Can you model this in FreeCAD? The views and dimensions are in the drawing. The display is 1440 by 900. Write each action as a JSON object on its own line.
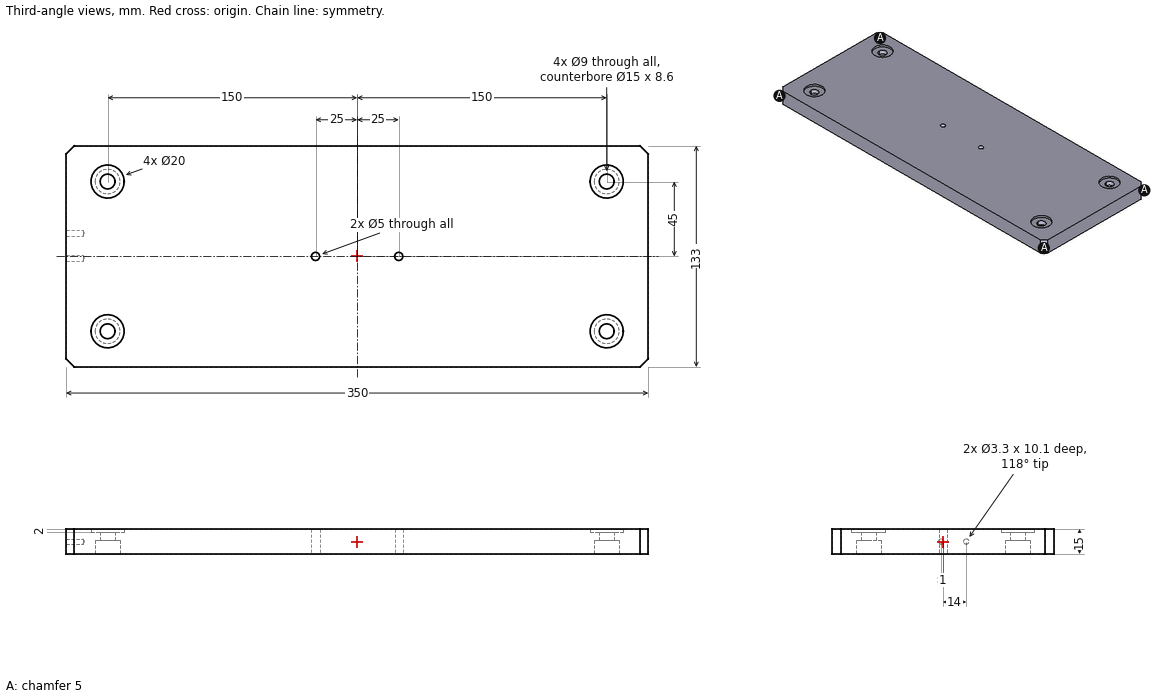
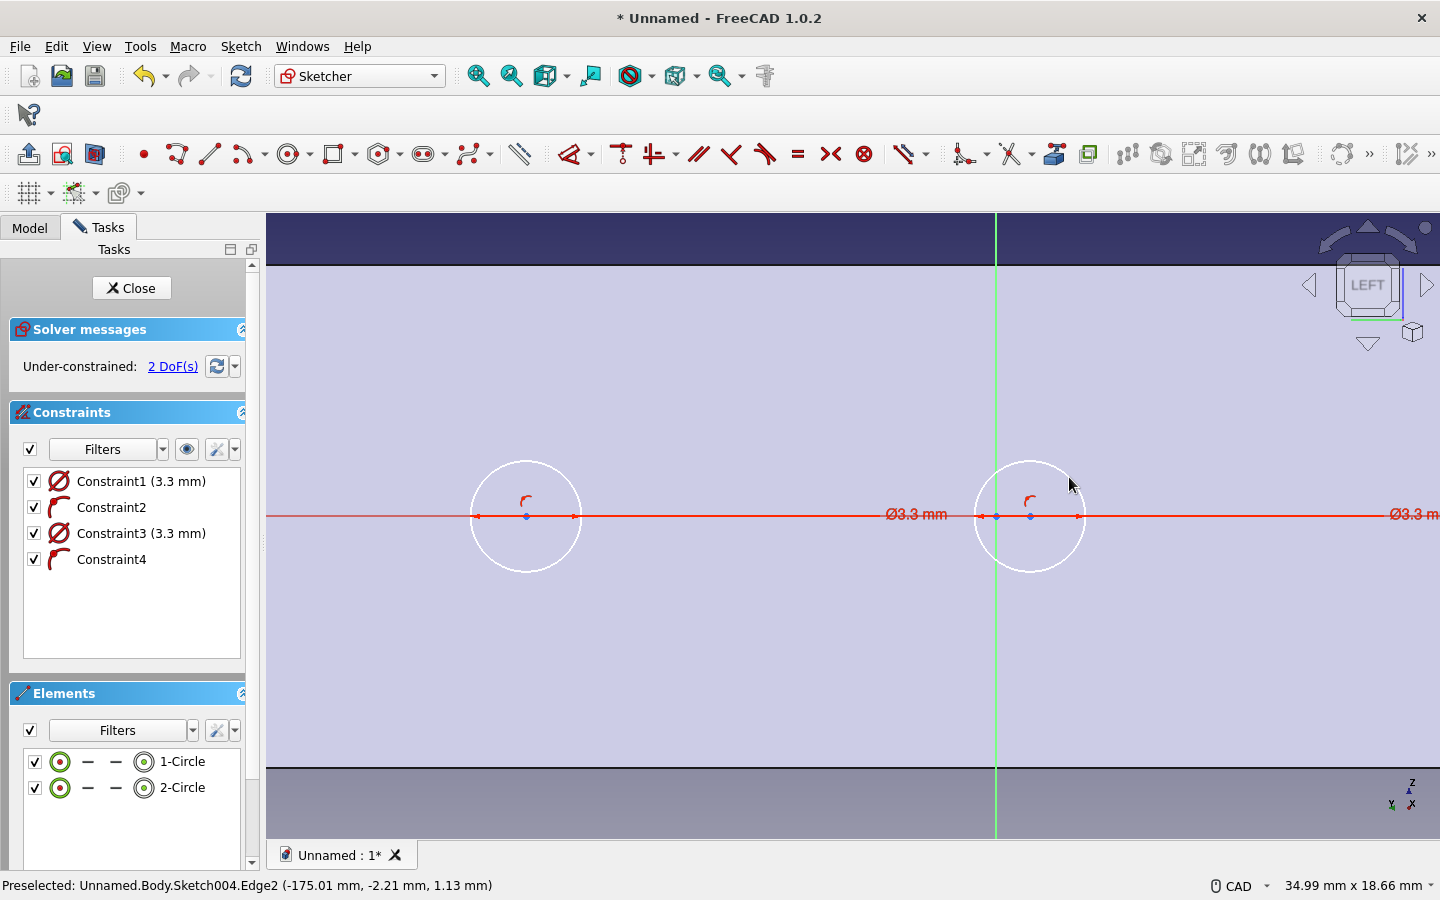
{"action": "left_click", "coordinate": [568, 154]}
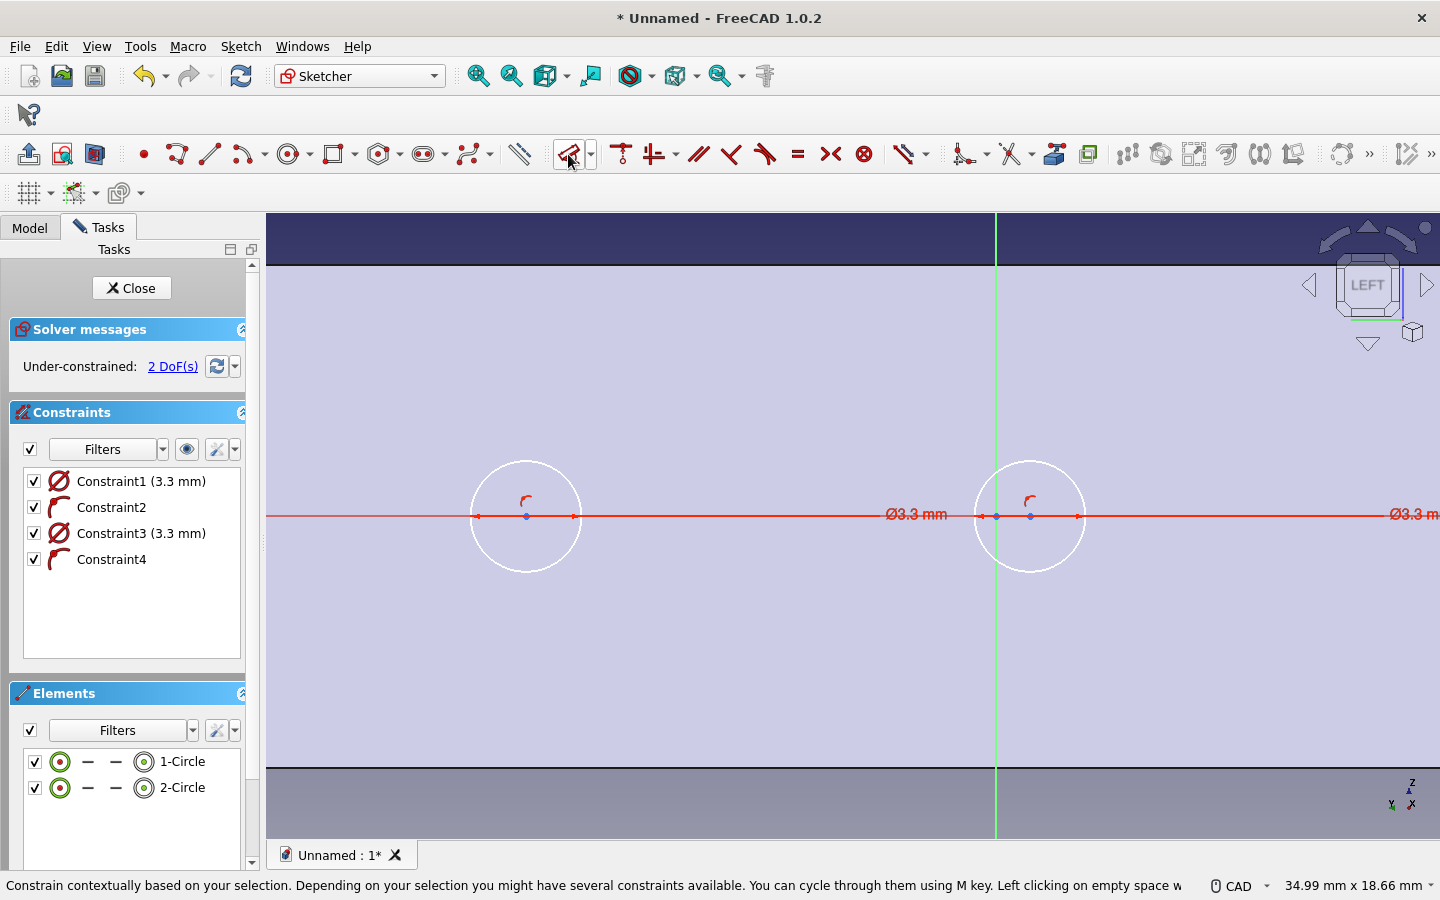
{"action": "left_click", "coordinate": [1030, 516]}
{"action": "left_click", "coordinate": [1013, 550]}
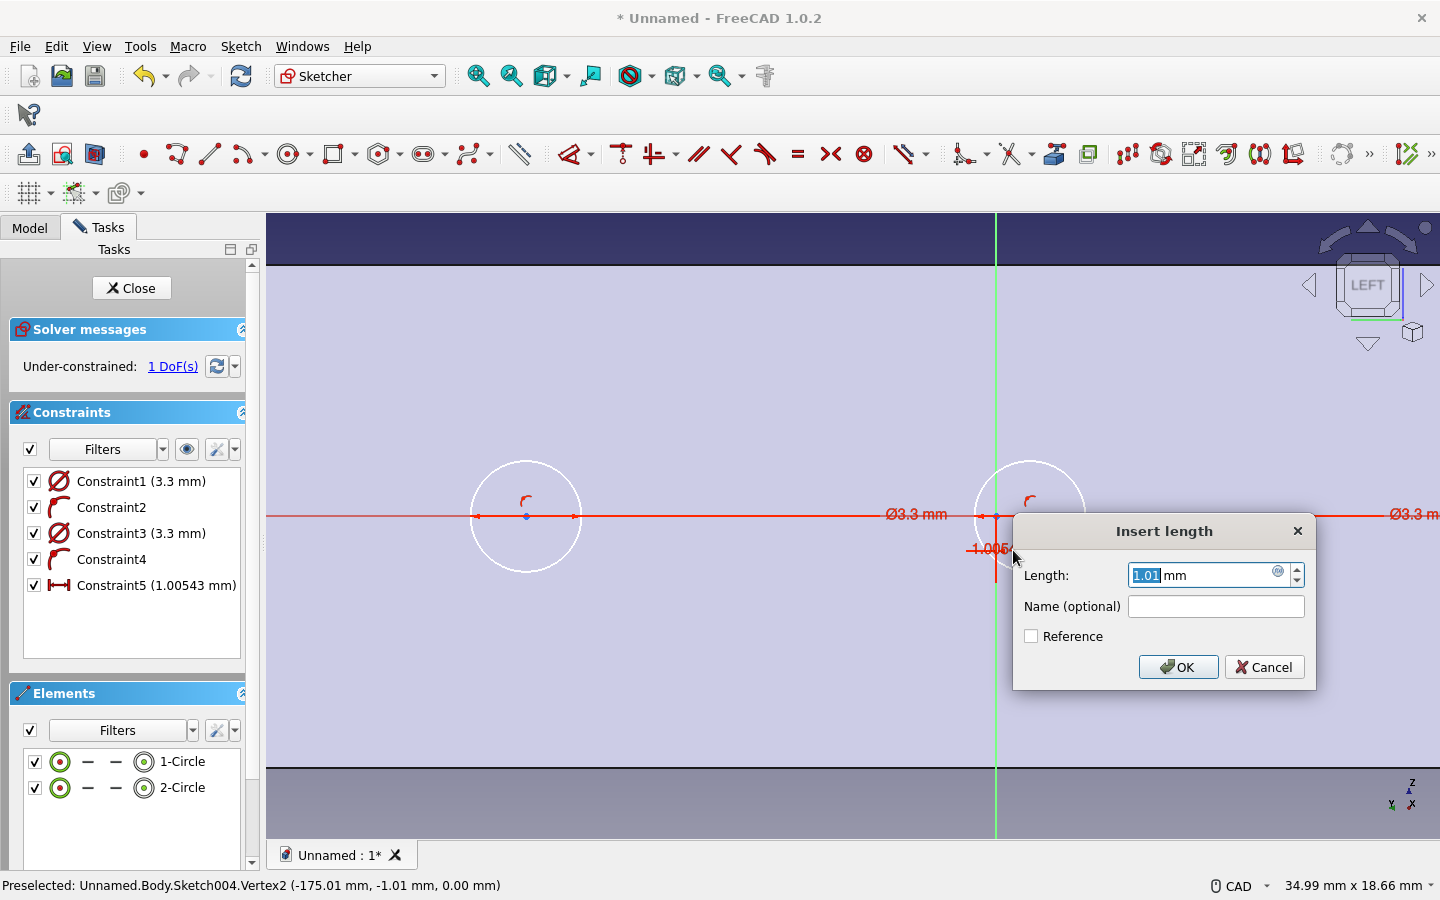
{"action": "type", "text": "1"}
{"action": "key", "text": "Return"}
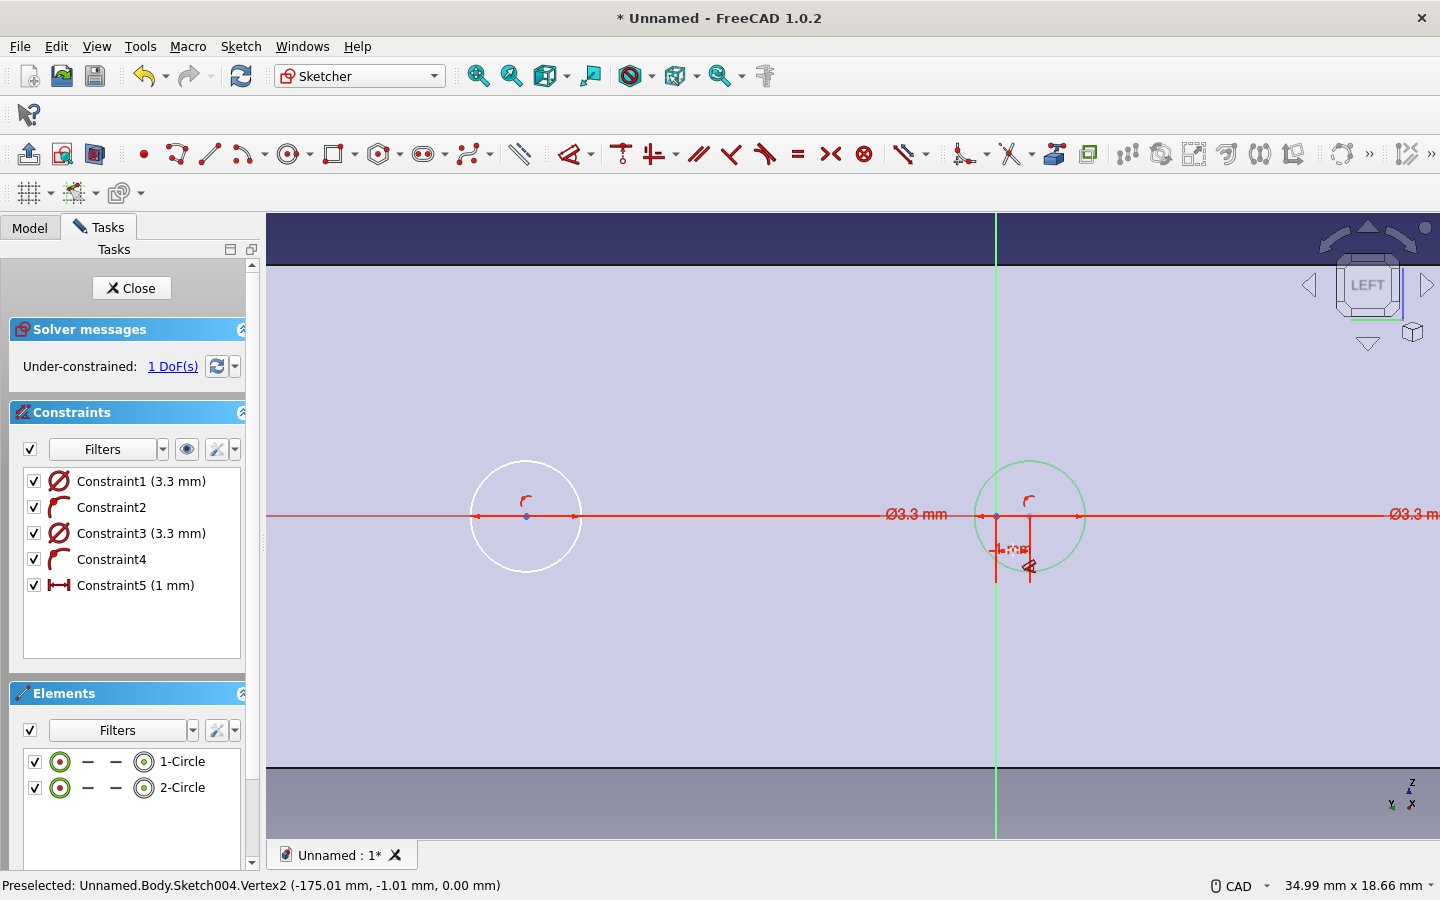
{"action": "left_click", "coordinate": [526, 516]}
{"action": "left_click", "coordinate": [761, 550]}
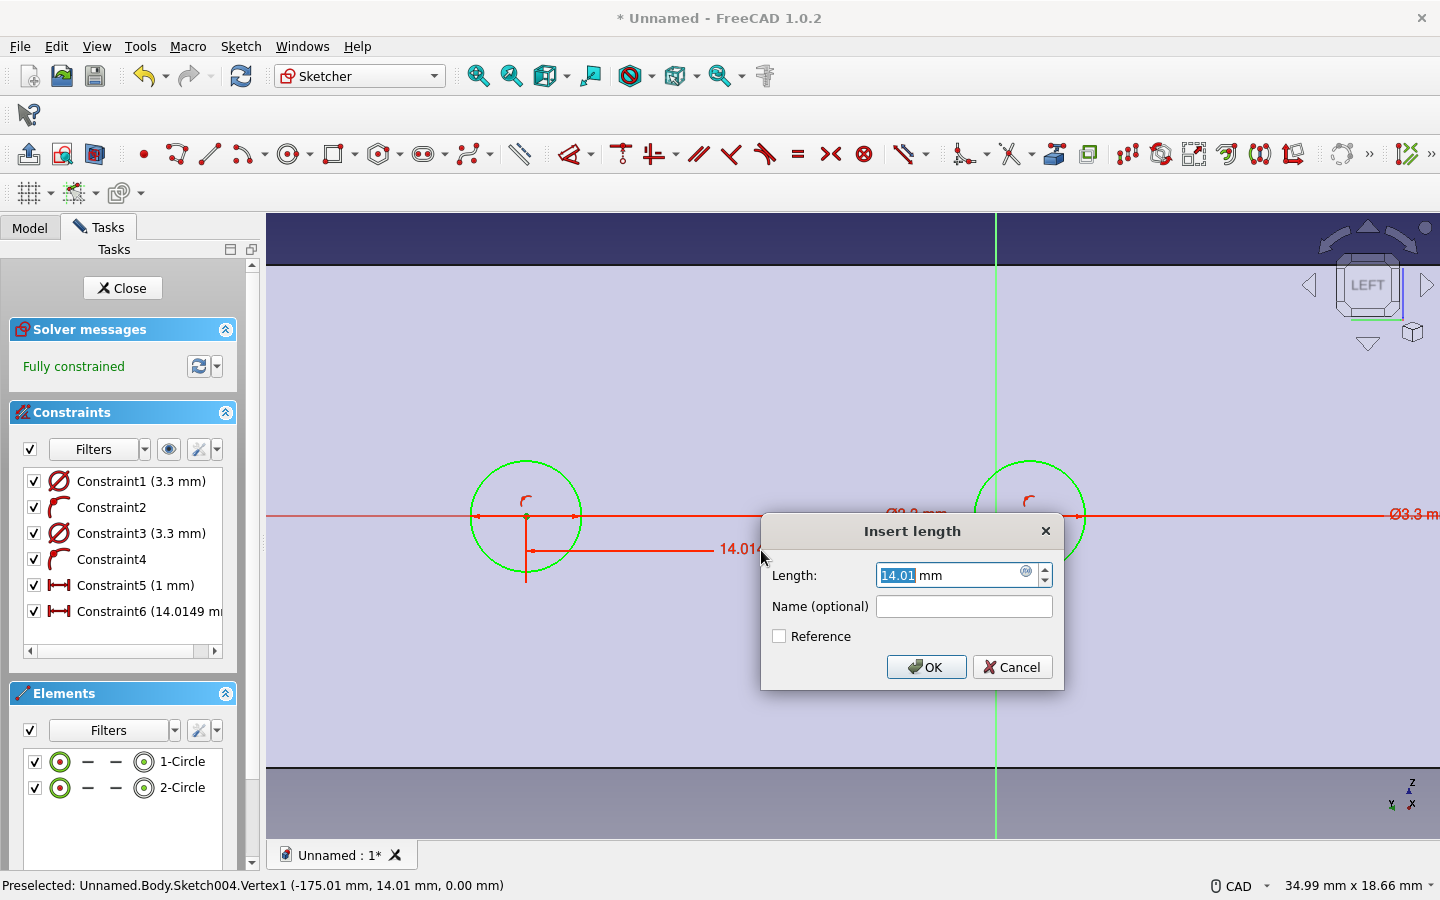
{"action": "type", "text": "14"}
{"action": "key", "text": "Return"}
{"action": "key", "text": "Escape"}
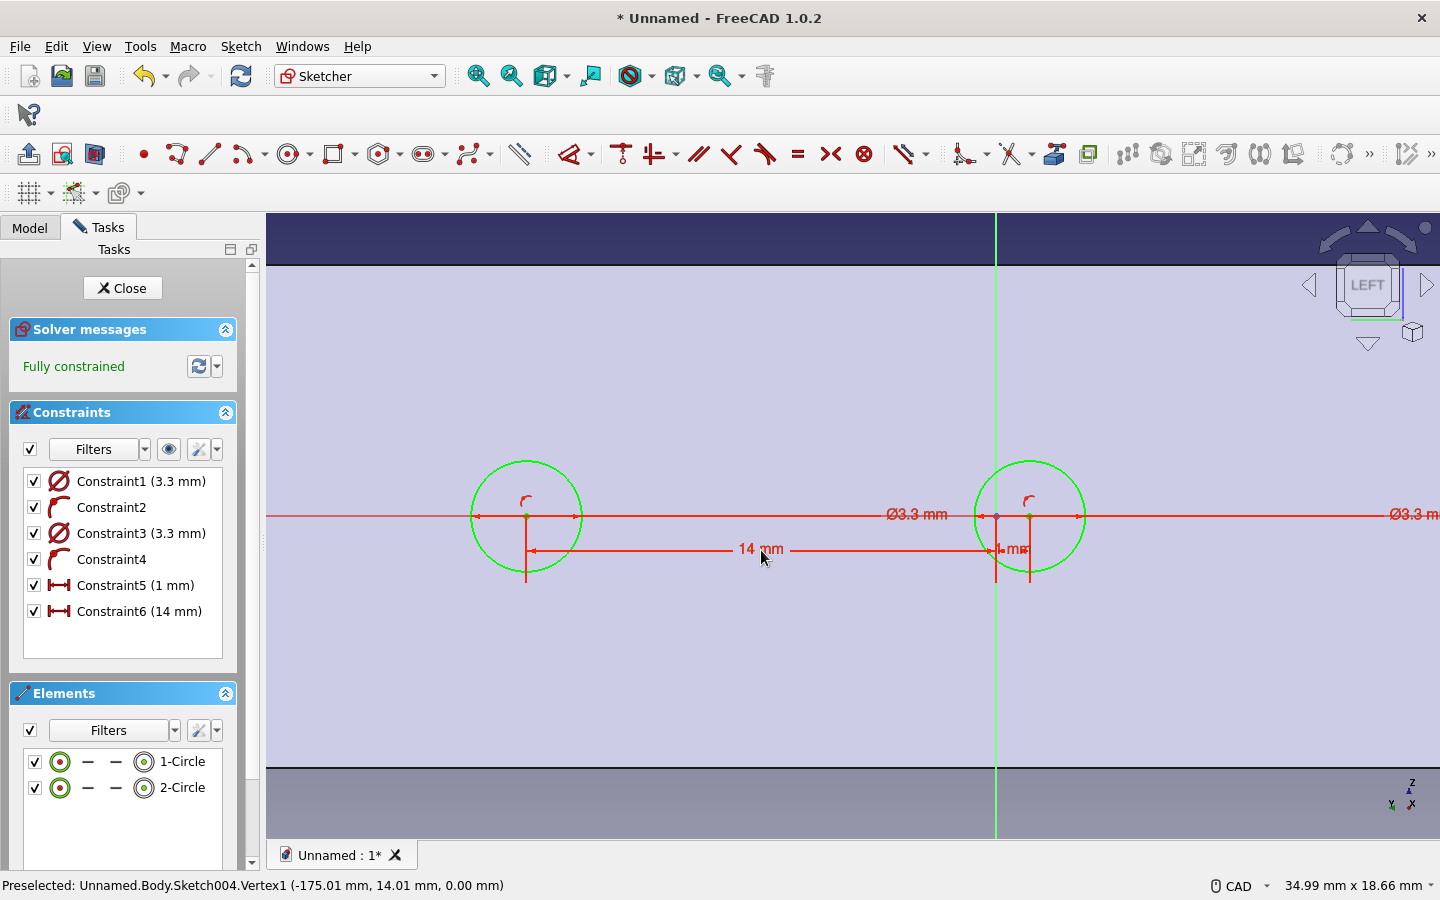
{"action": "left_click", "coordinate": [123, 288]}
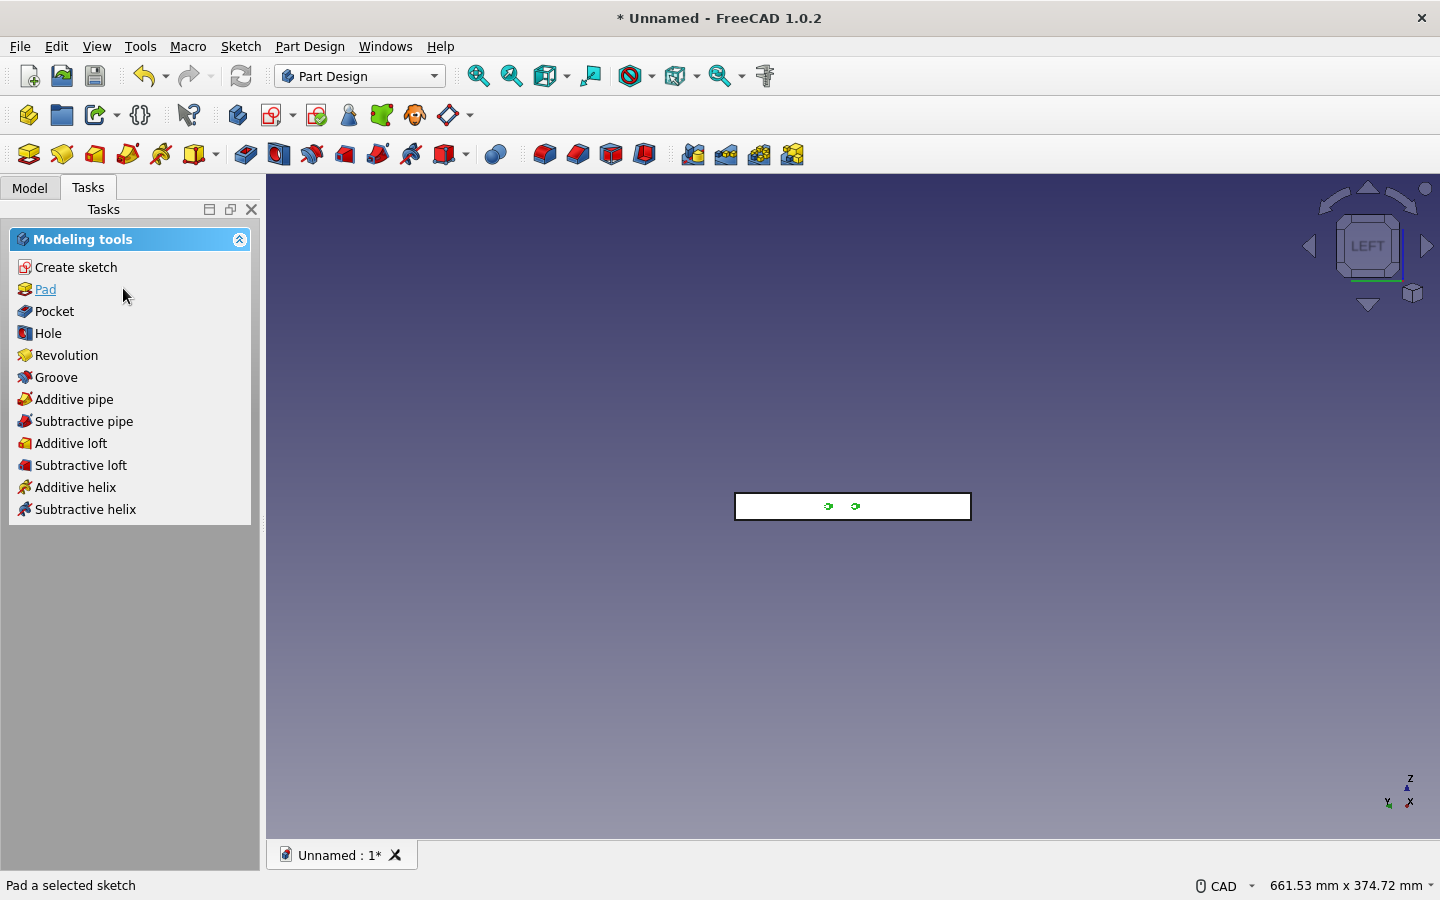
{"action": "left_click", "coordinate": [279, 154]}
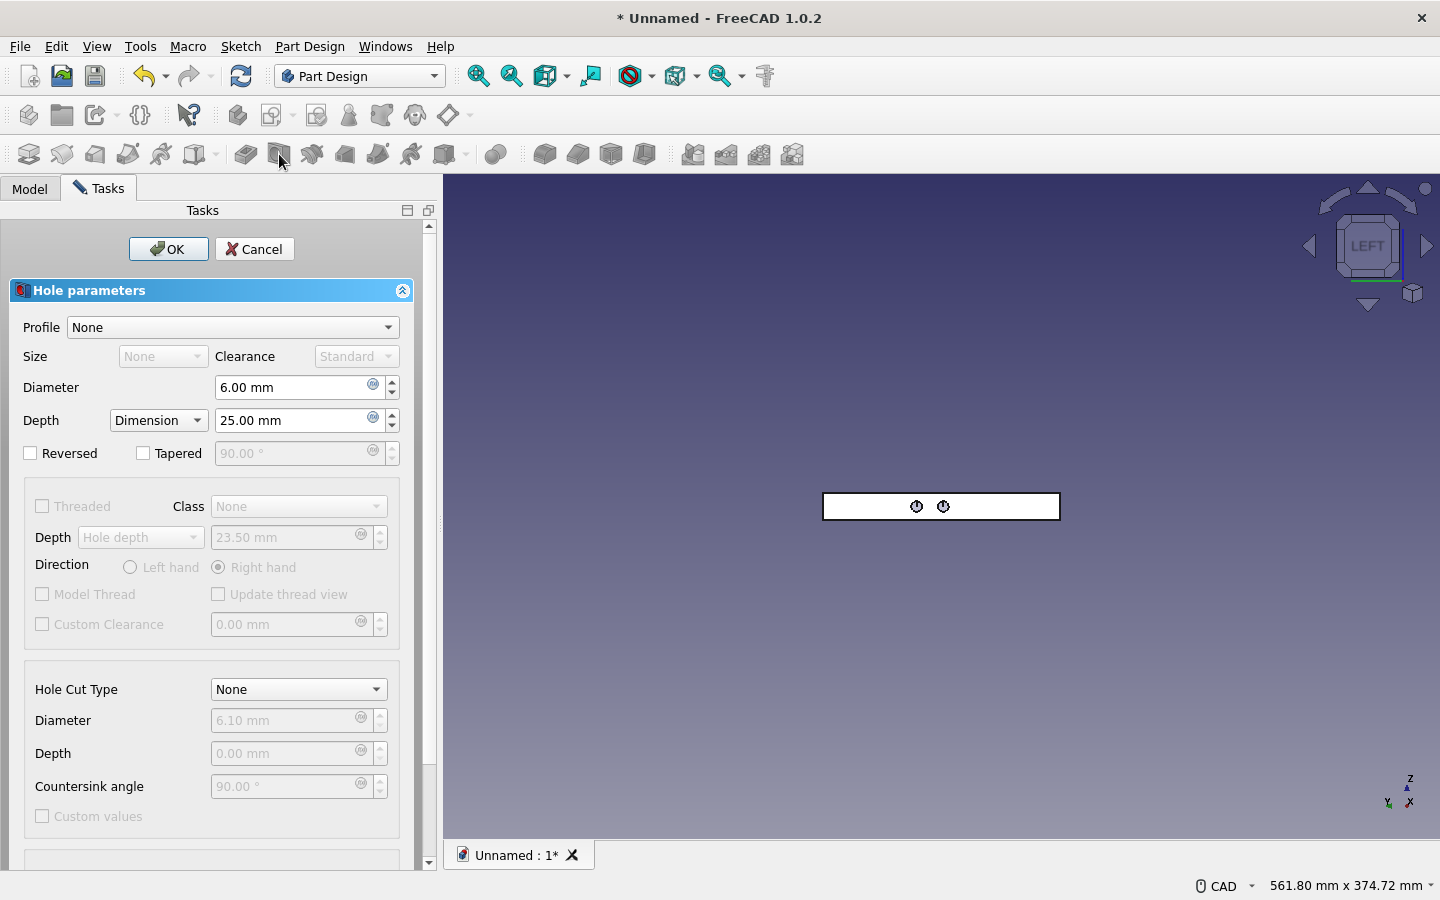
{"action": "triple_click", "coordinate": [300, 388]}